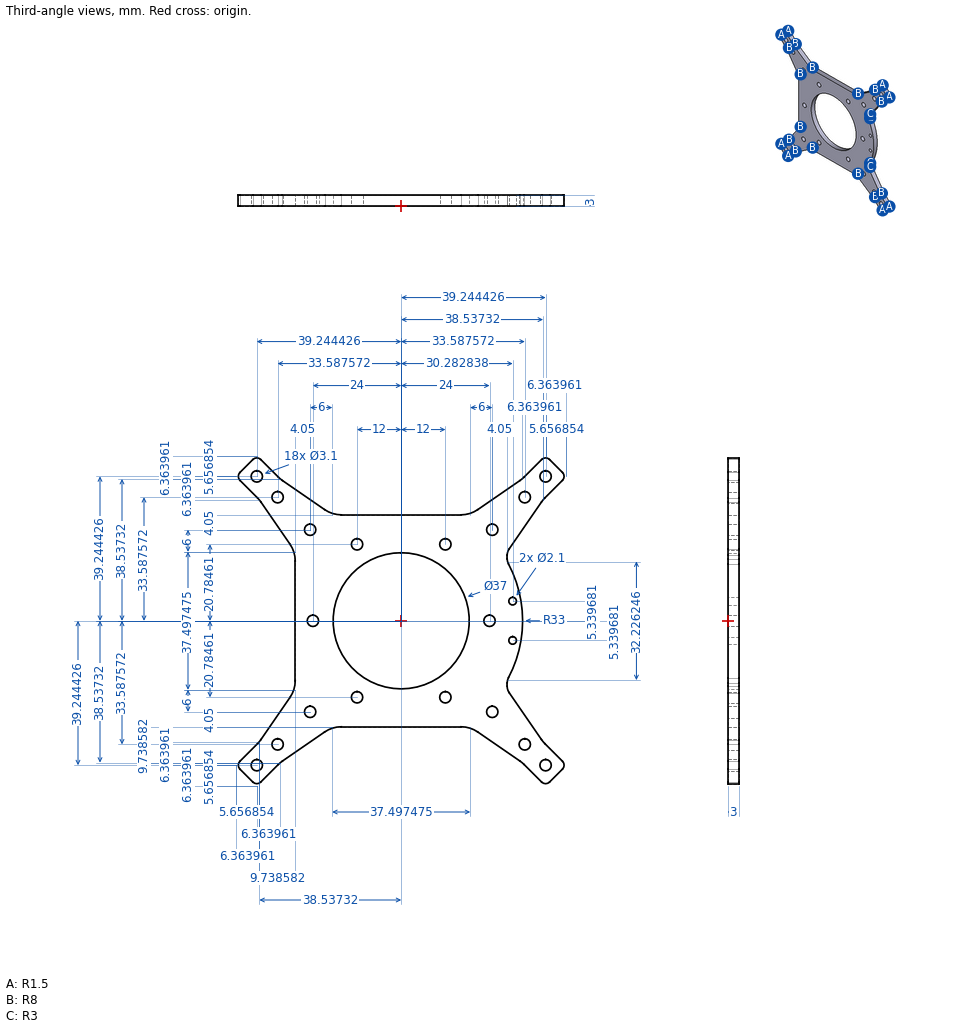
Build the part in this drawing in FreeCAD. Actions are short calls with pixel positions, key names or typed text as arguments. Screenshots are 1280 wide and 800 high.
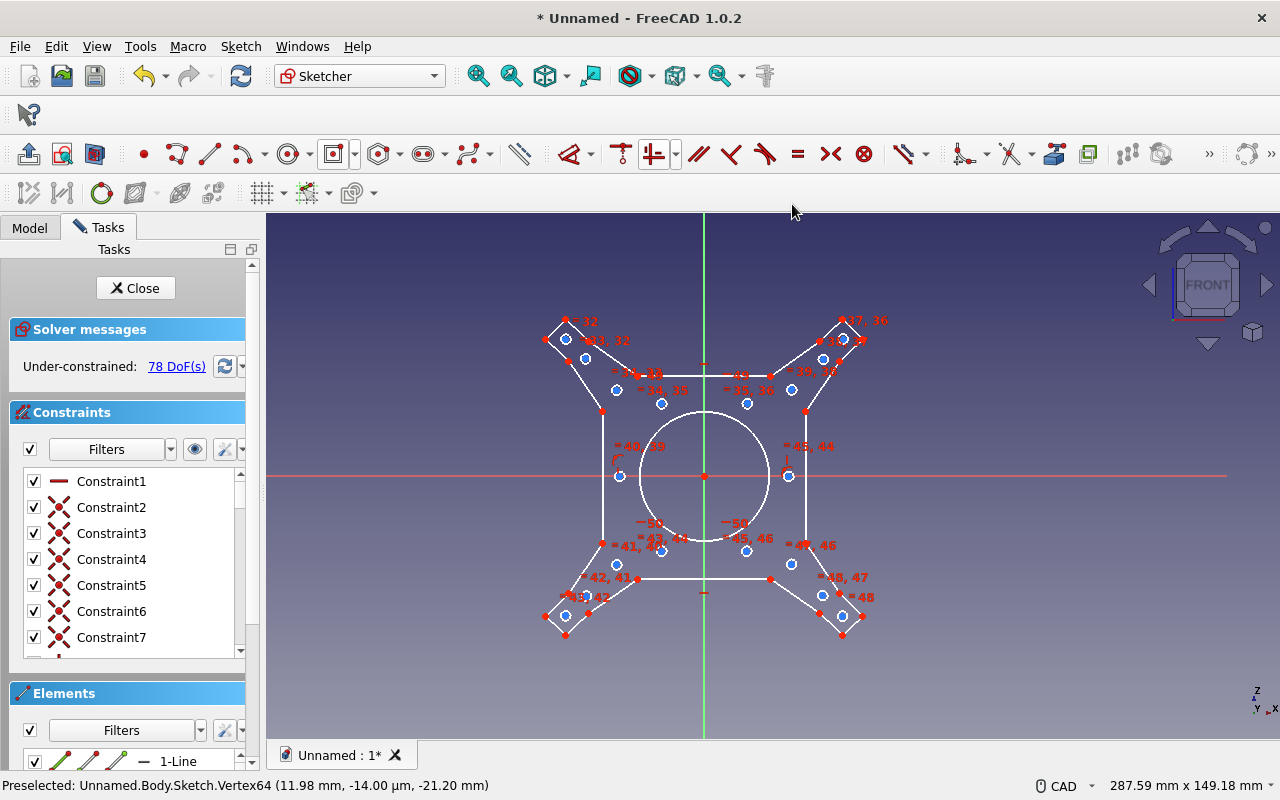
scroll(569, 336, up, 7)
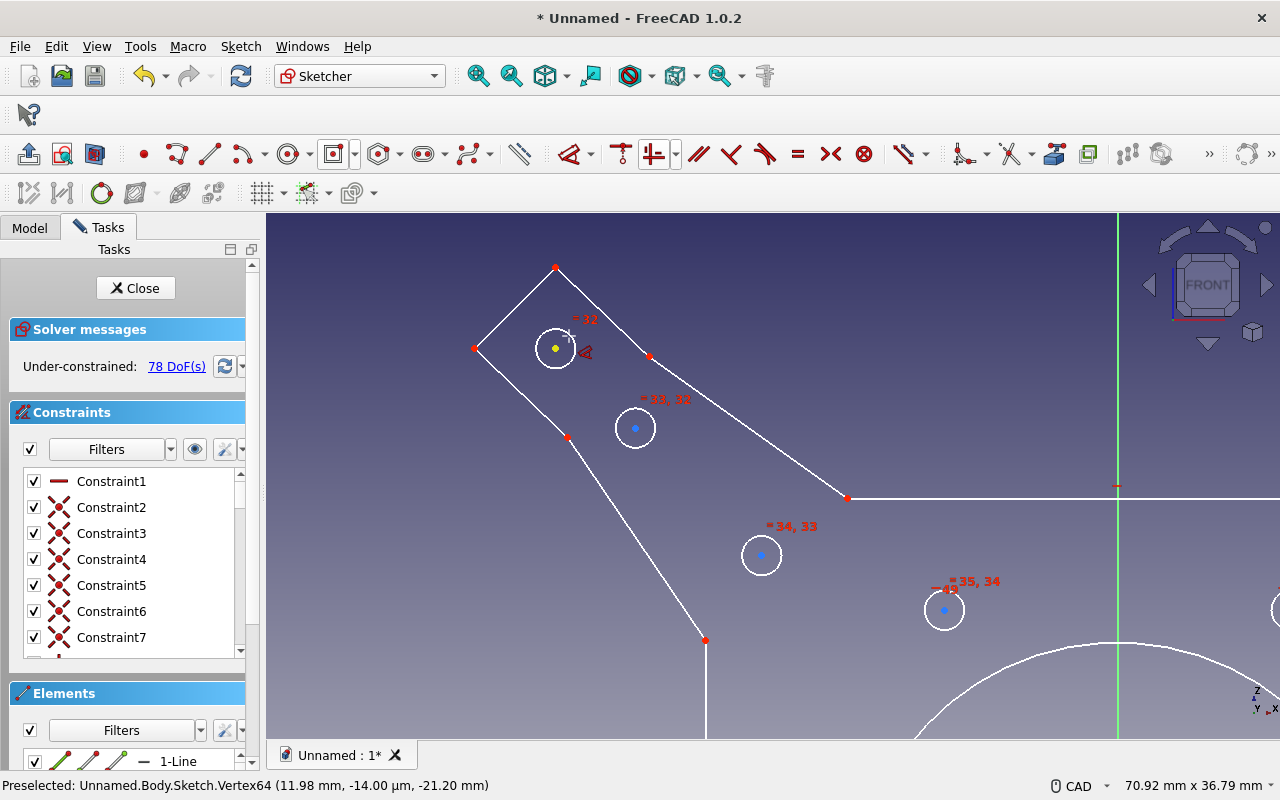
click(570, 335)
click(606, 335)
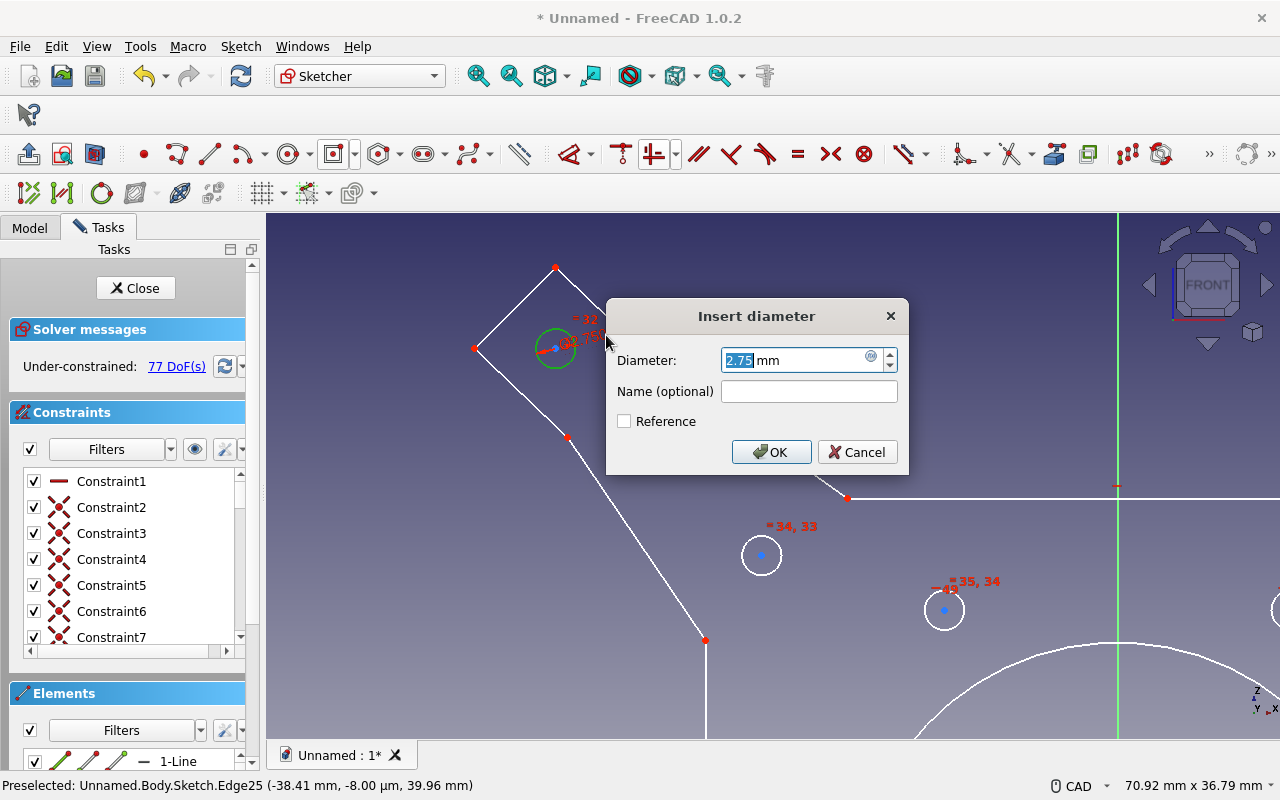
text(3.1)
key(Return)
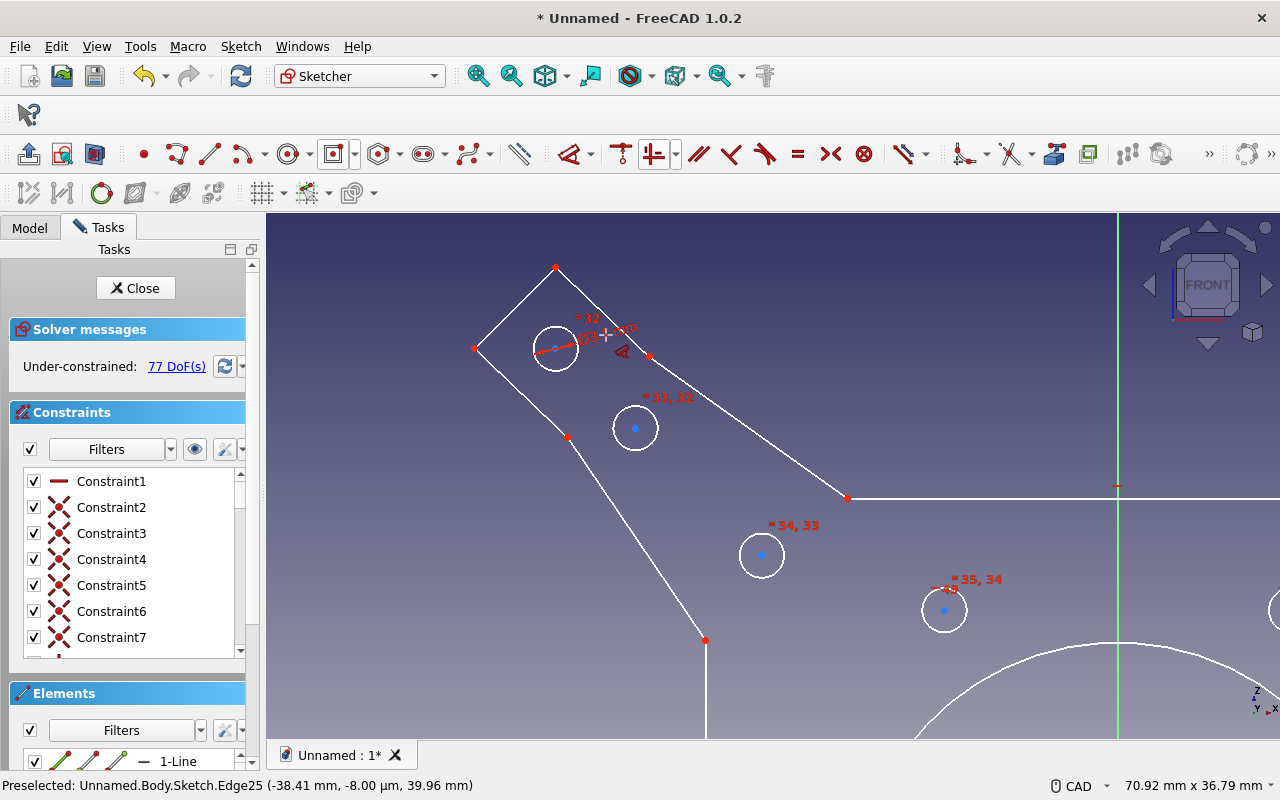
scroll(569, 336, down, 7)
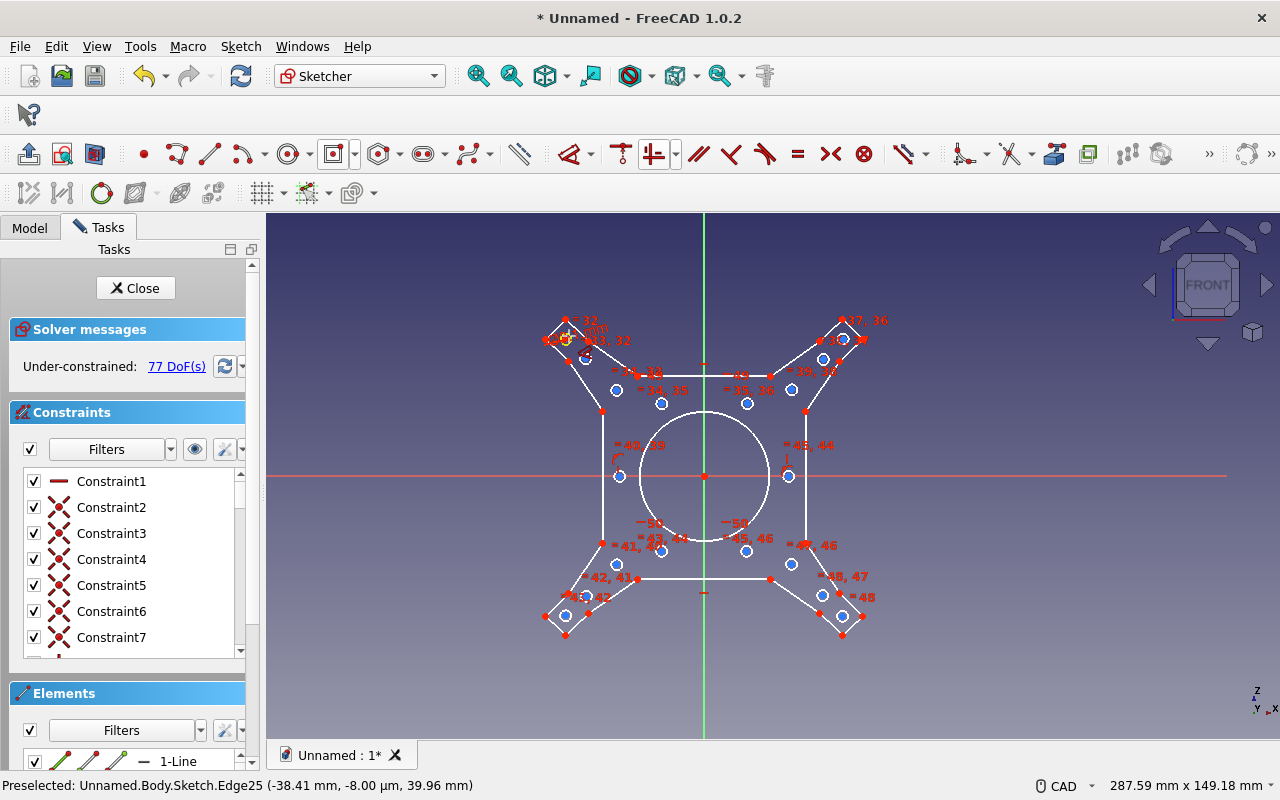
click(750, 431)
click(773, 408)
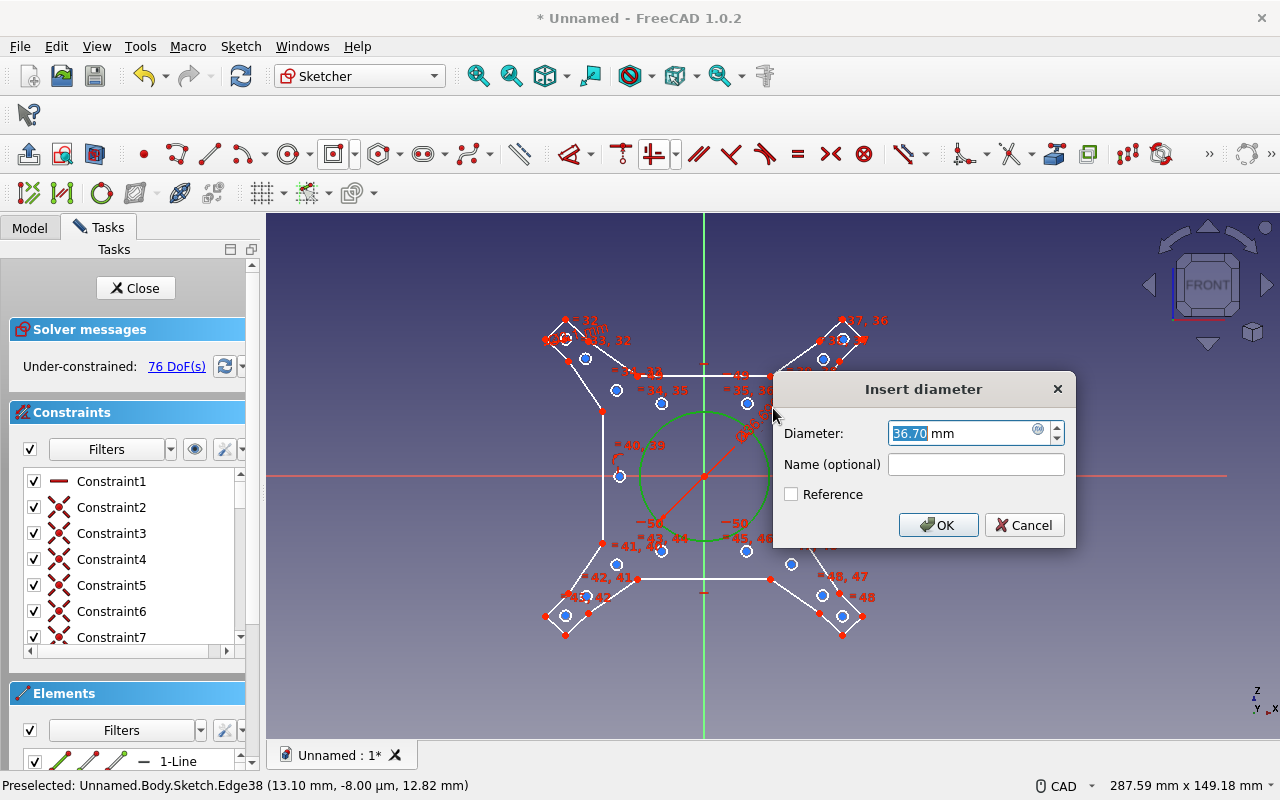
text(37)
key(Return)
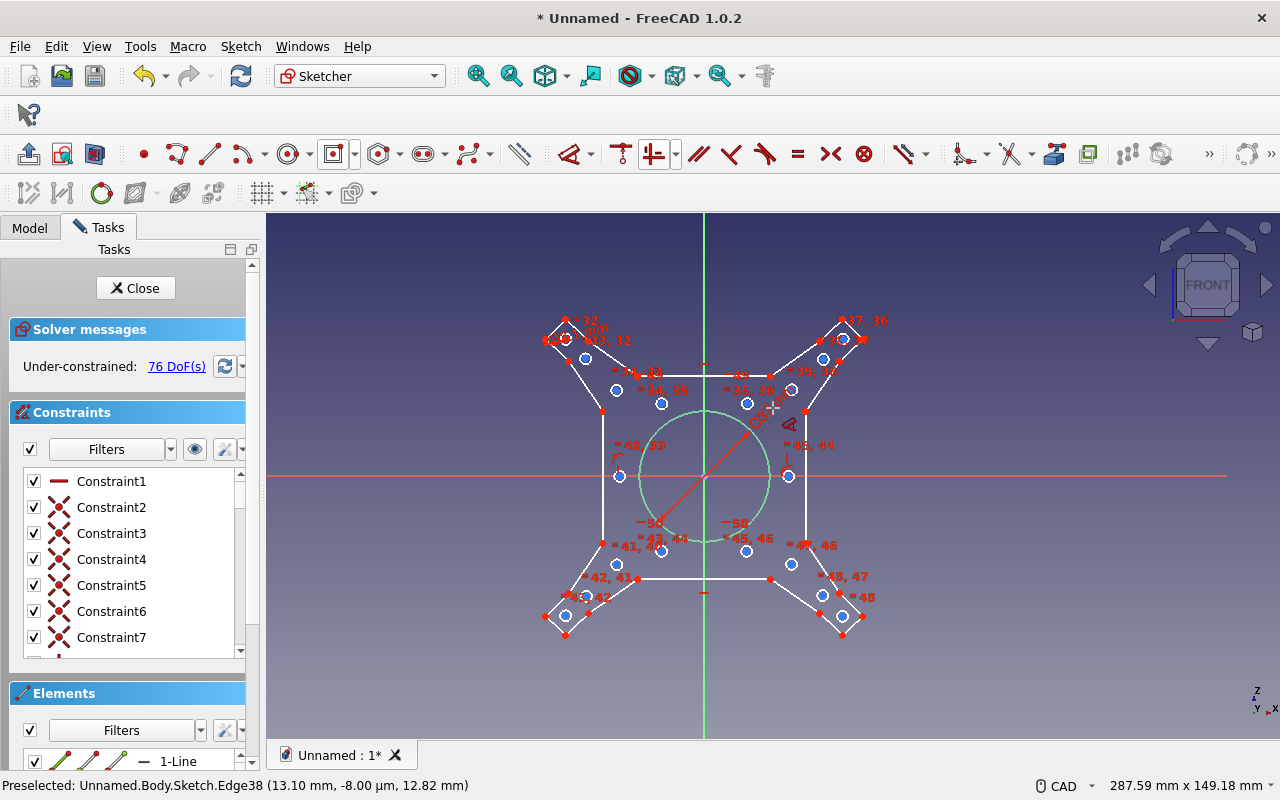
click(662, 404)
click(683, 510)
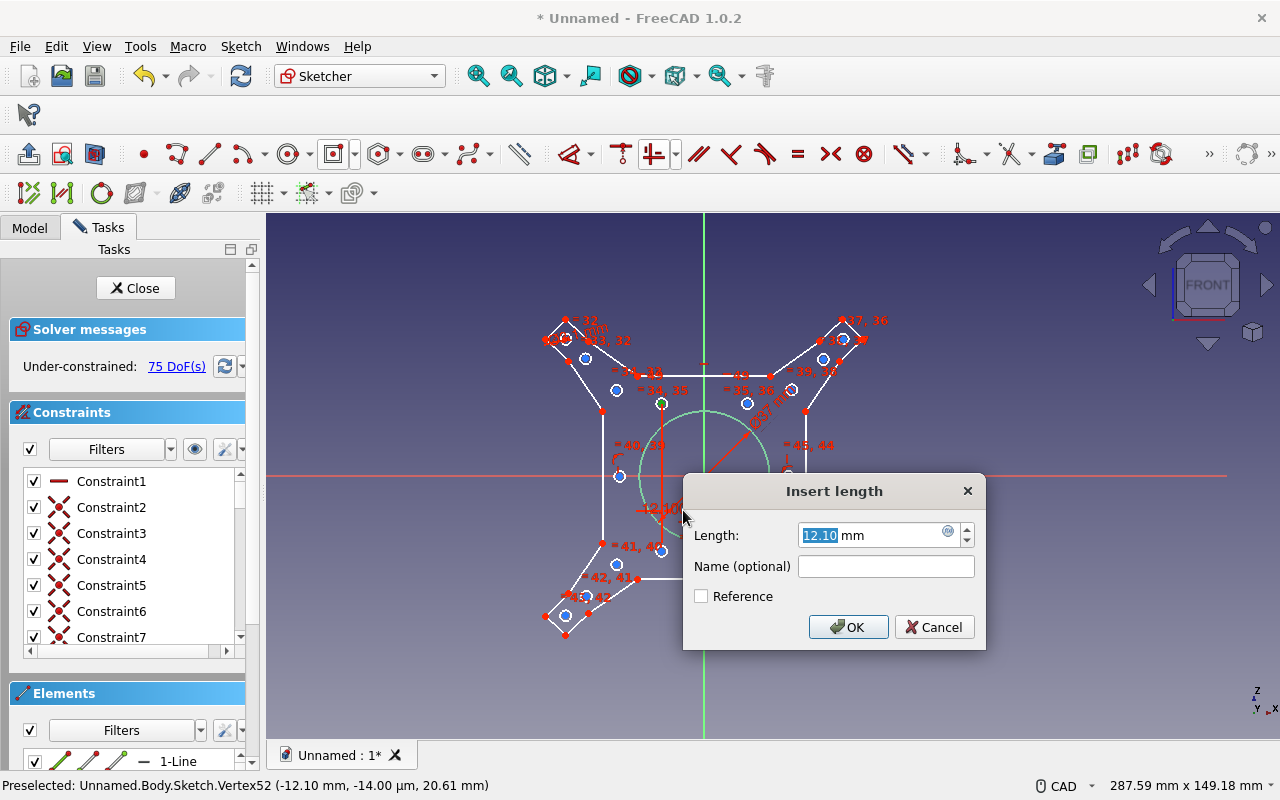
text(12)
key(Return)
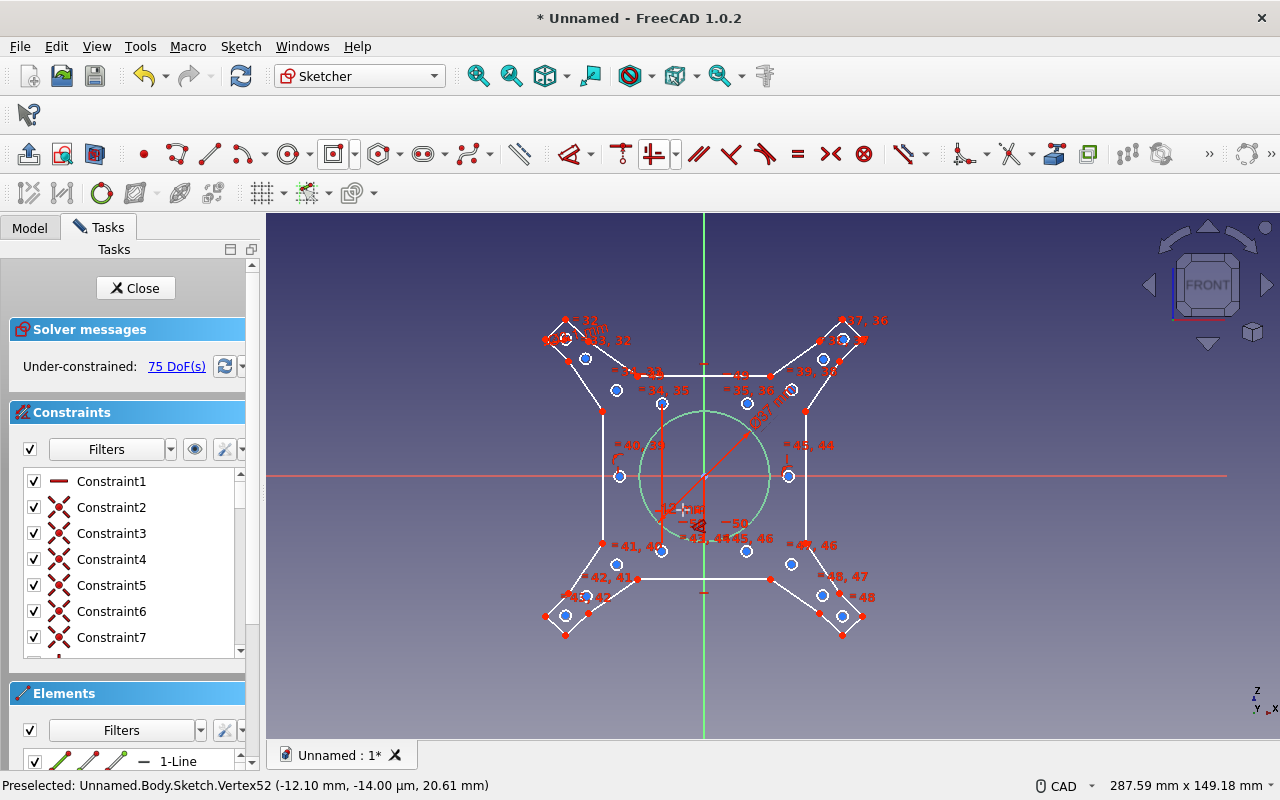
click(747, 404)
click(726, 346)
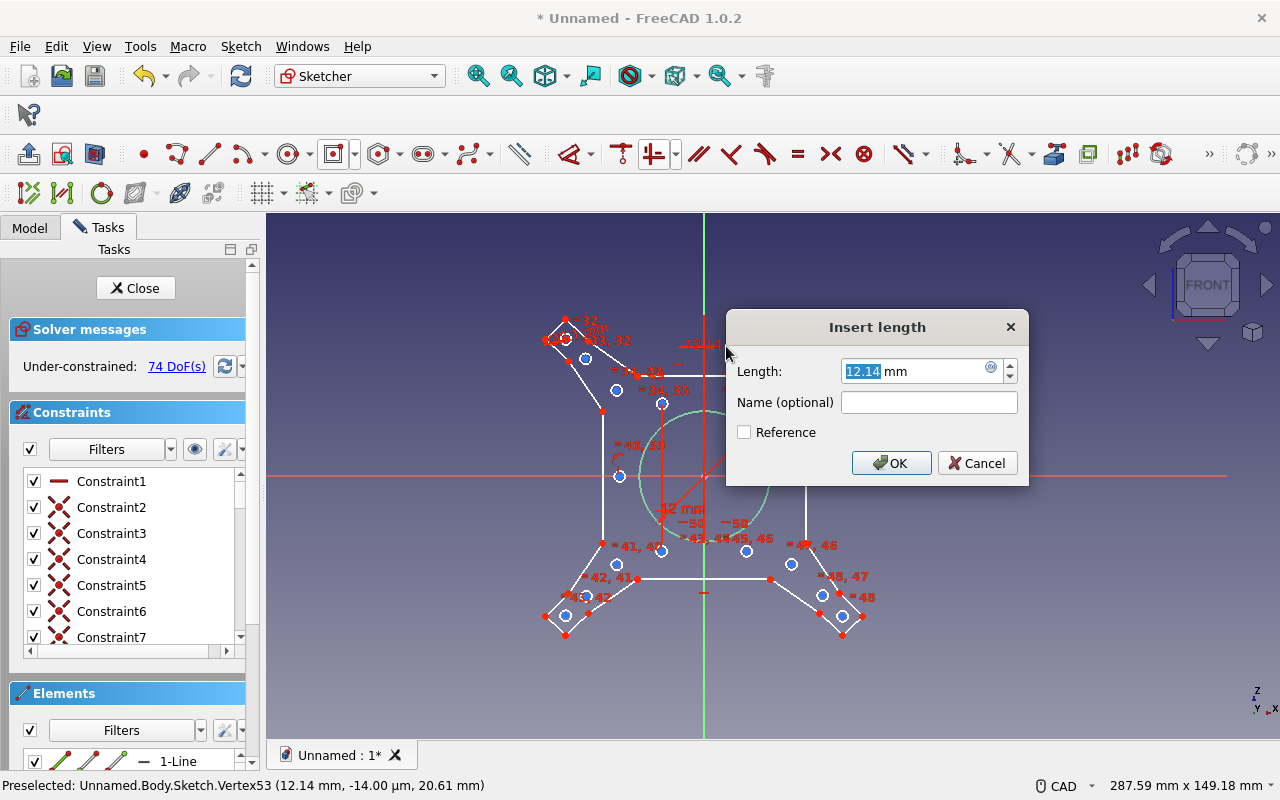
text(12)
key(Return)